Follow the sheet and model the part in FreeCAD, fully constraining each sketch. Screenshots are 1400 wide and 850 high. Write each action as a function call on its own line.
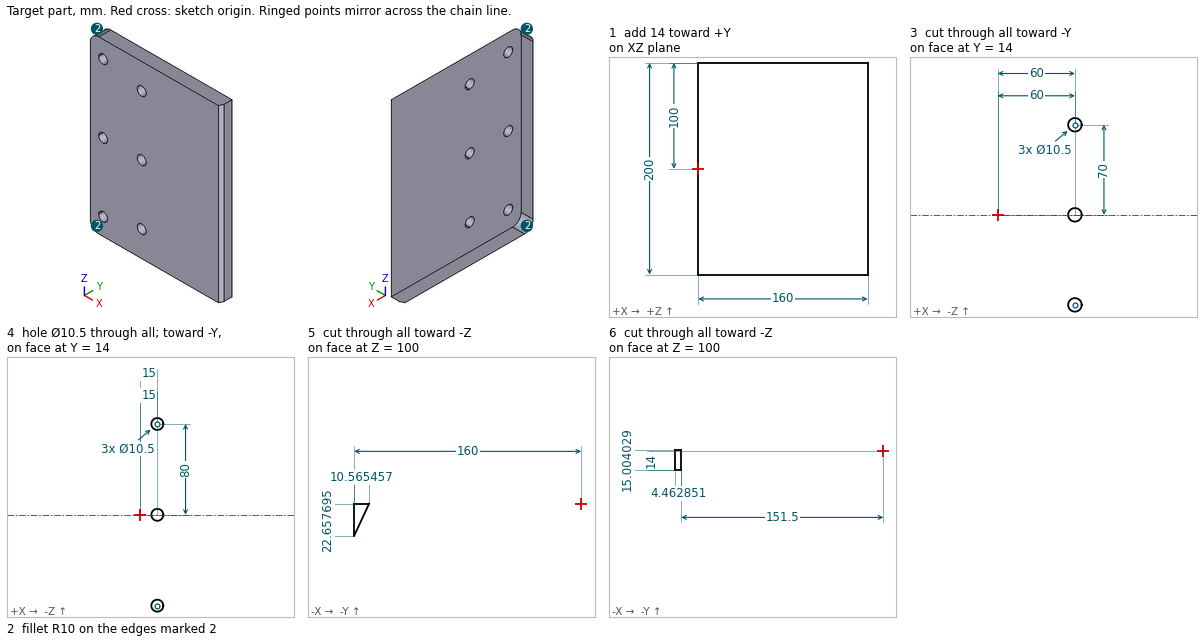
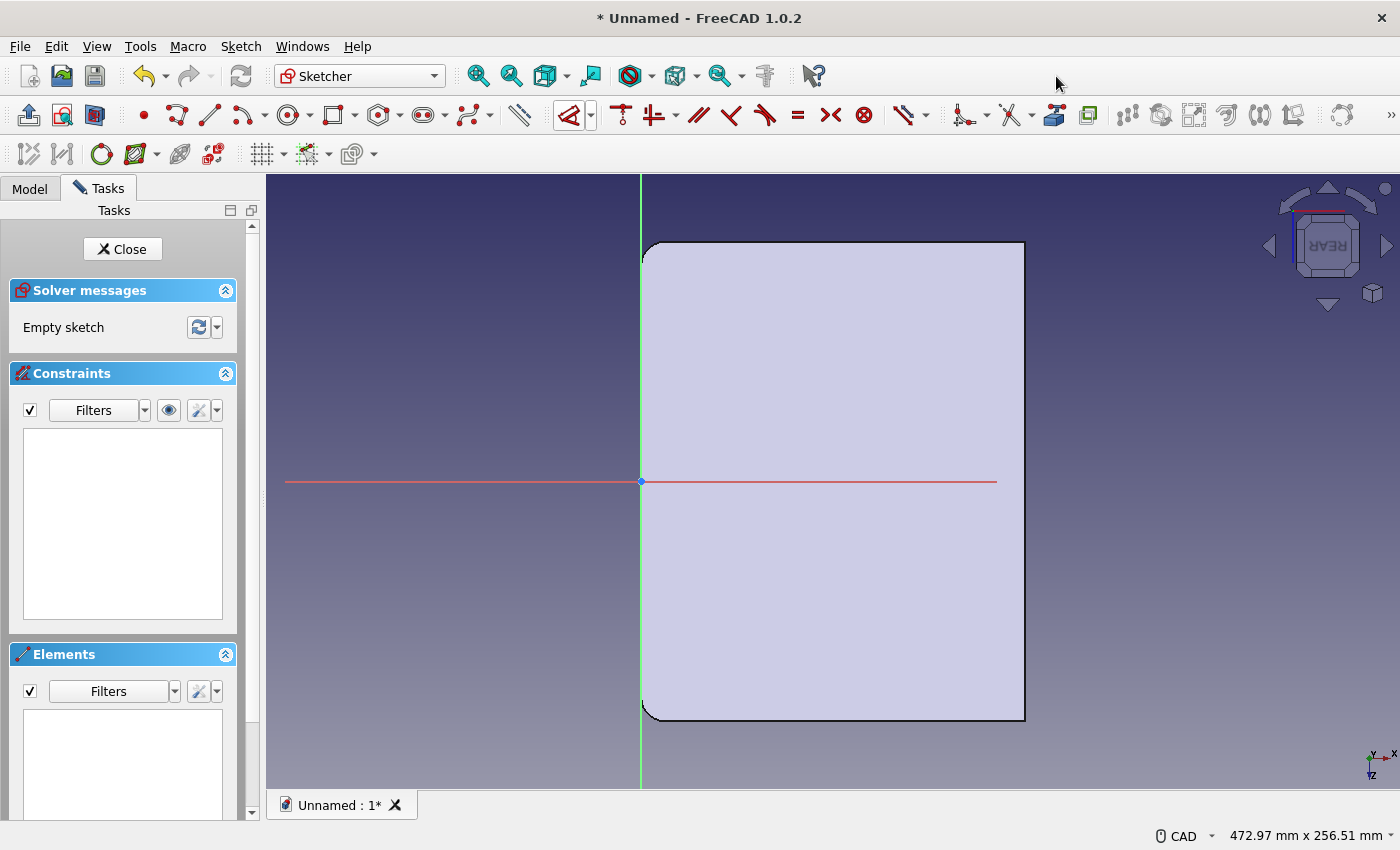
click(288, 116)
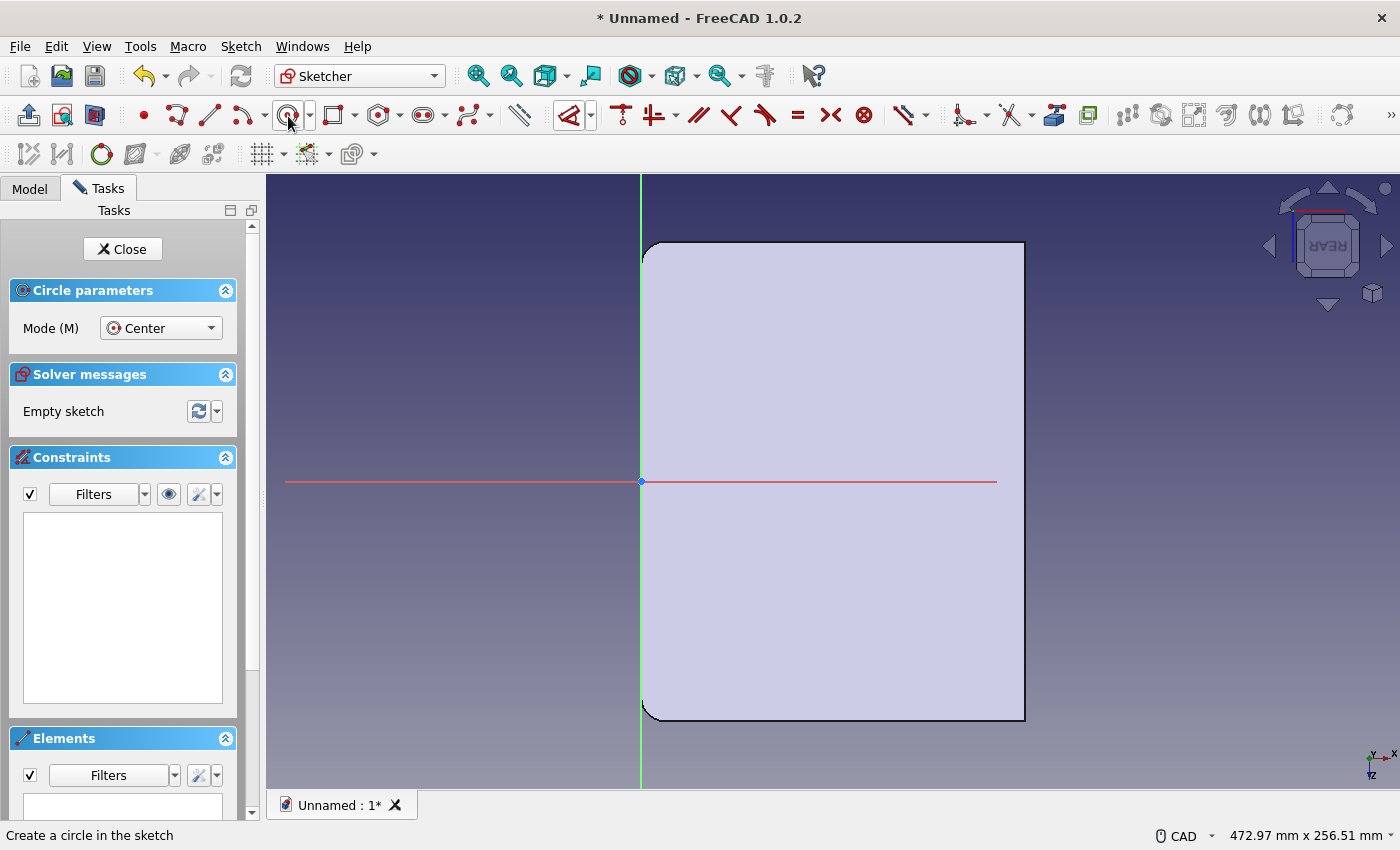
scroll(785, 314, up, 3)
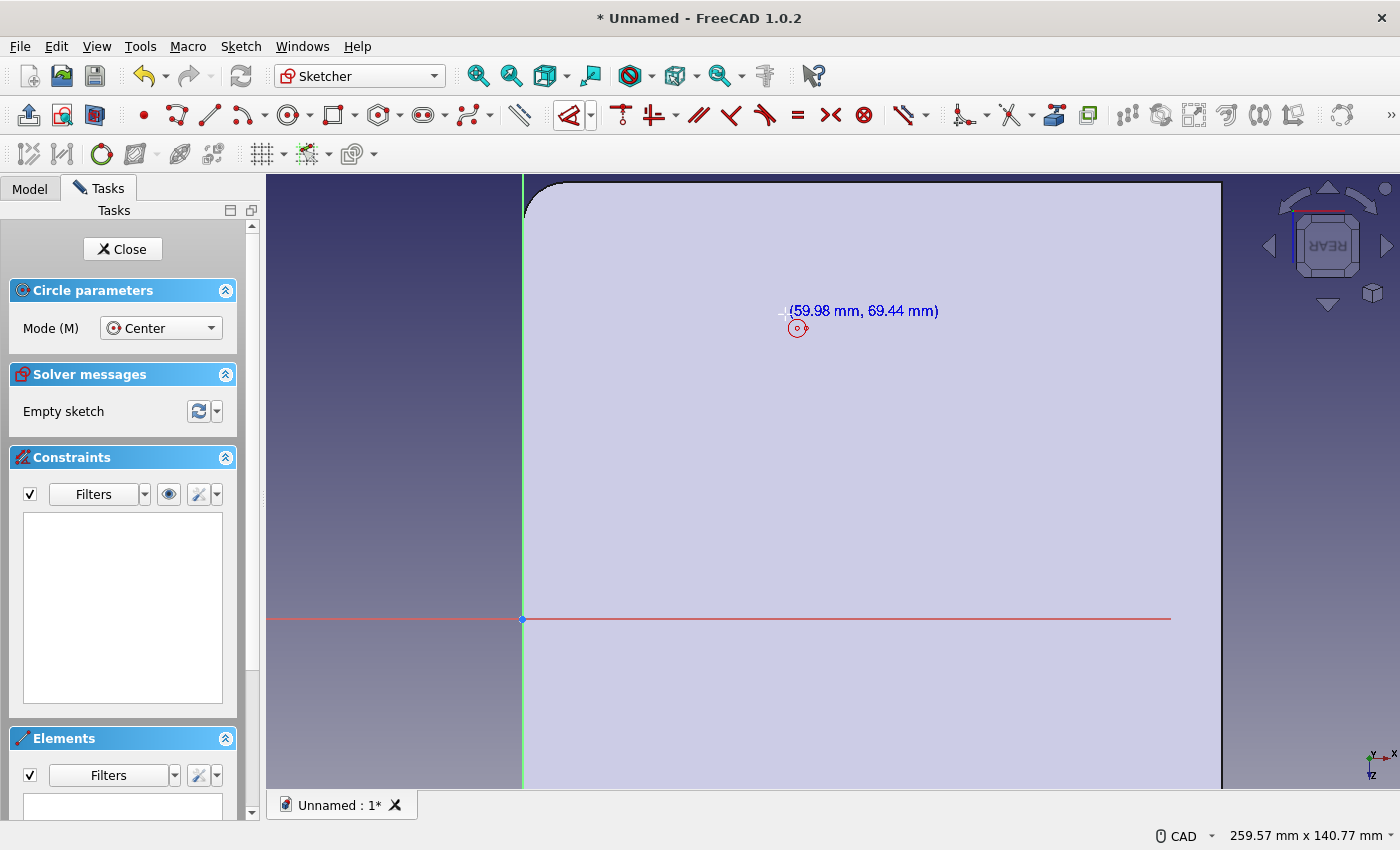
click(785, 313)
click(801, 297)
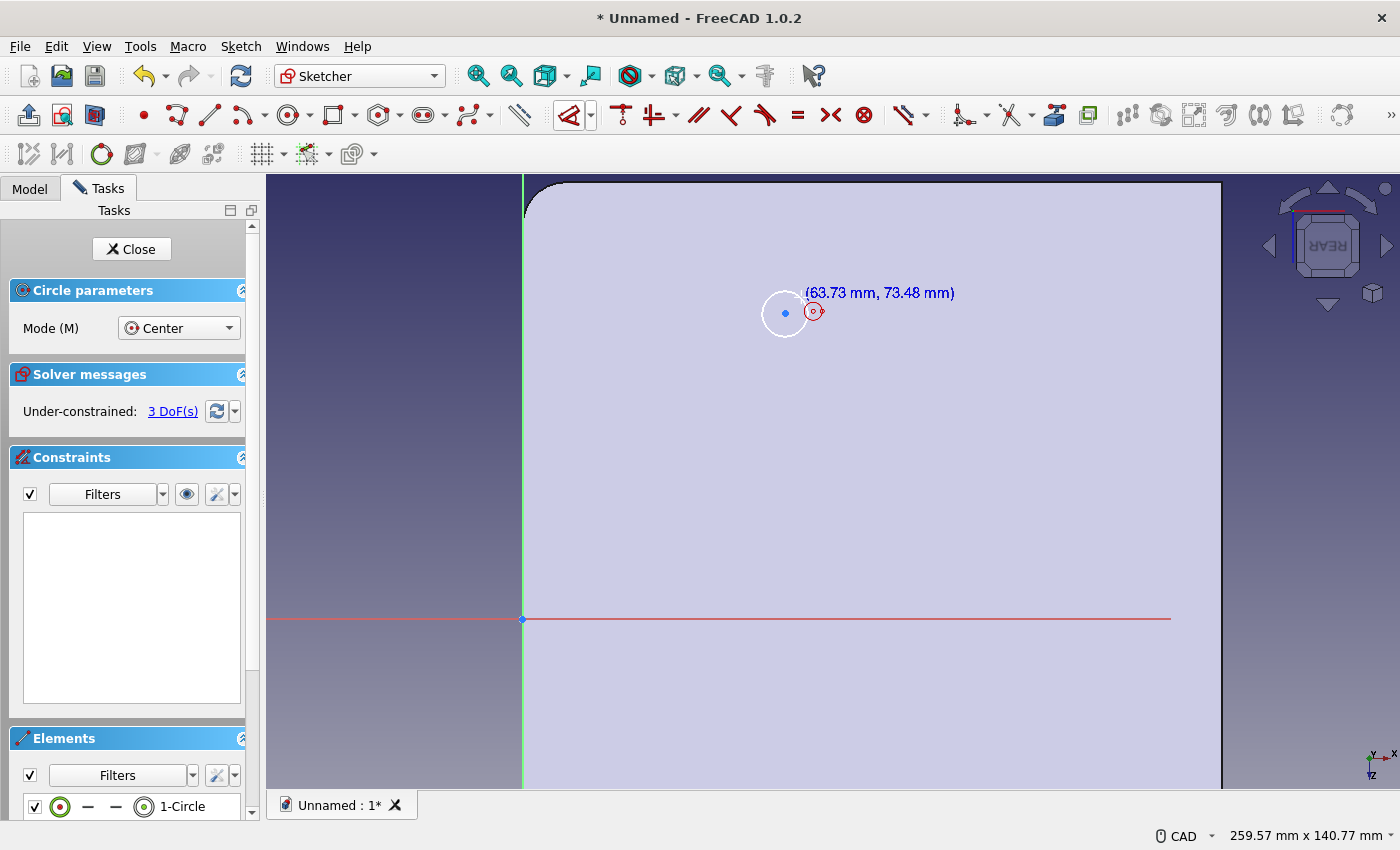
scroll(885, 314, down, 3)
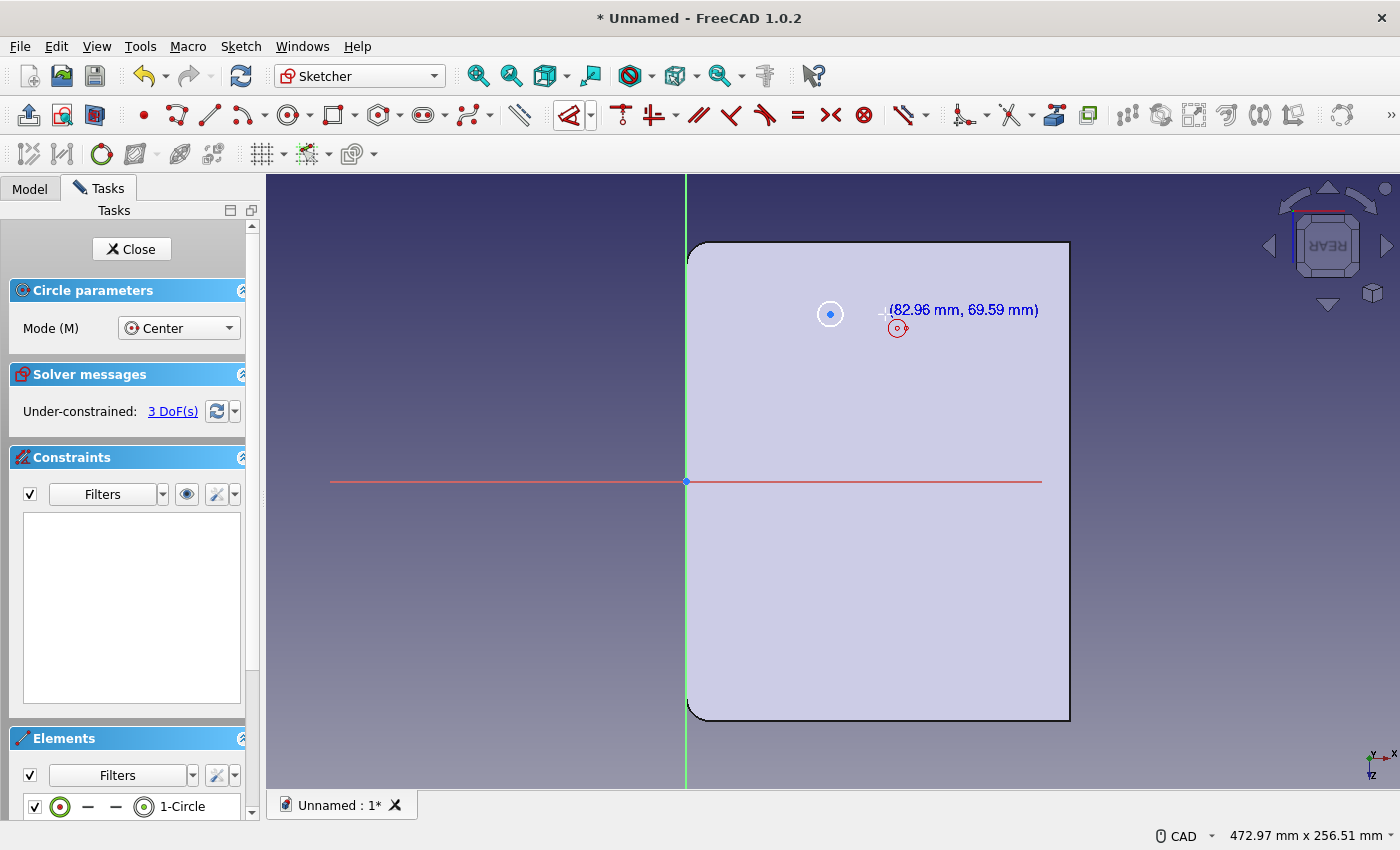
scroll(830, 649, up, 3)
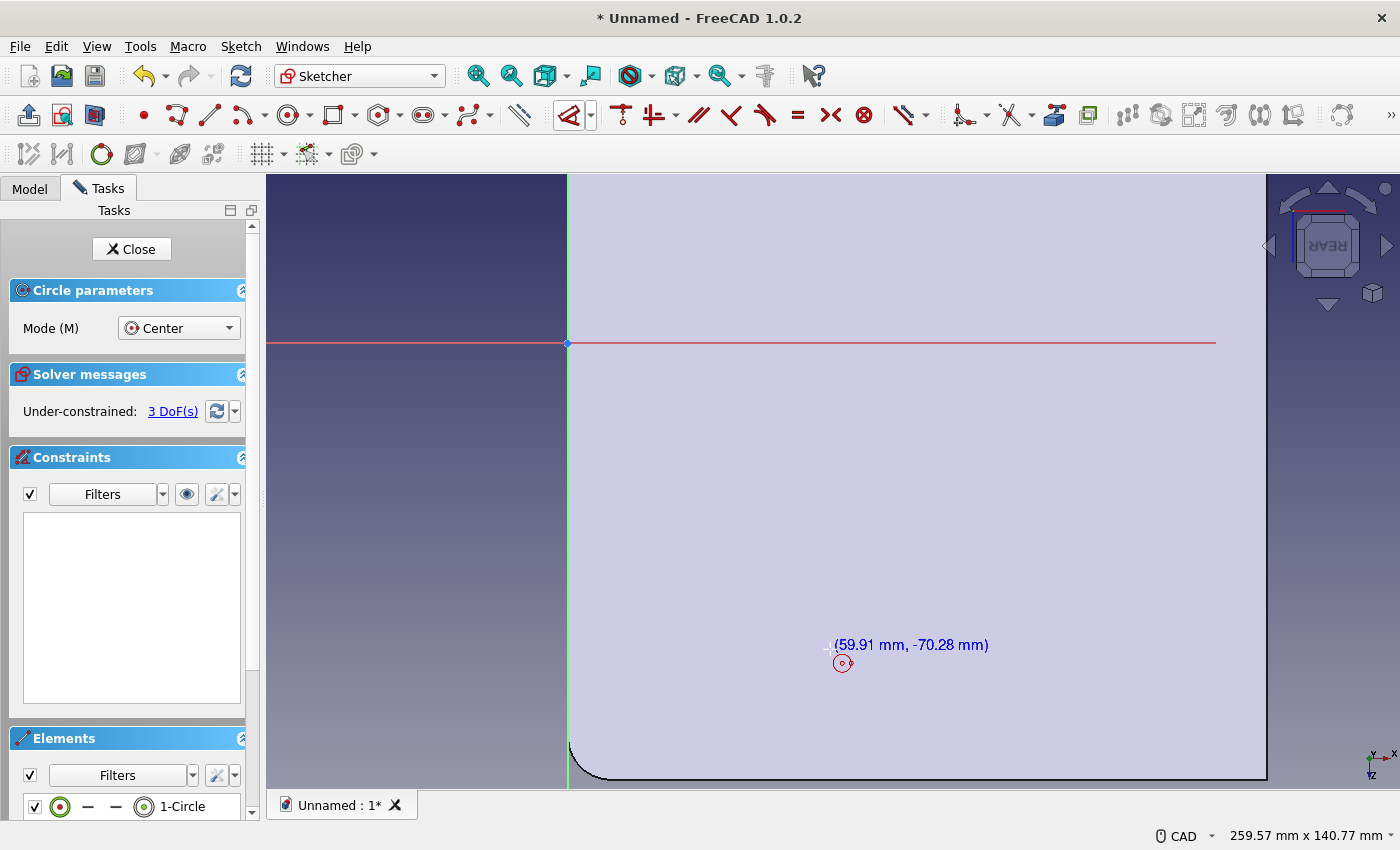
click(830, 649)
click(846, 633)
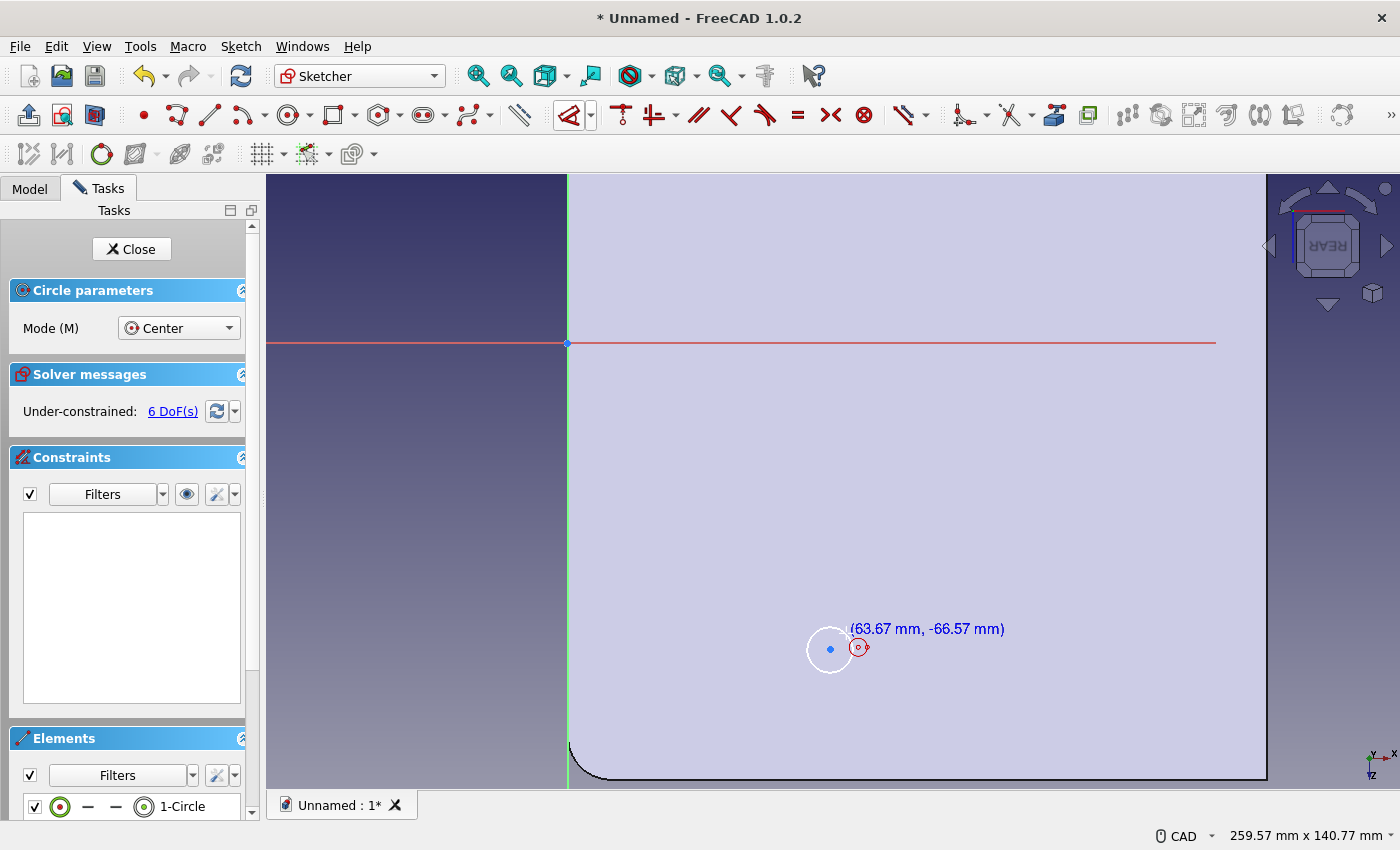
click(830, 343)
click(846, 327)
key(Escape)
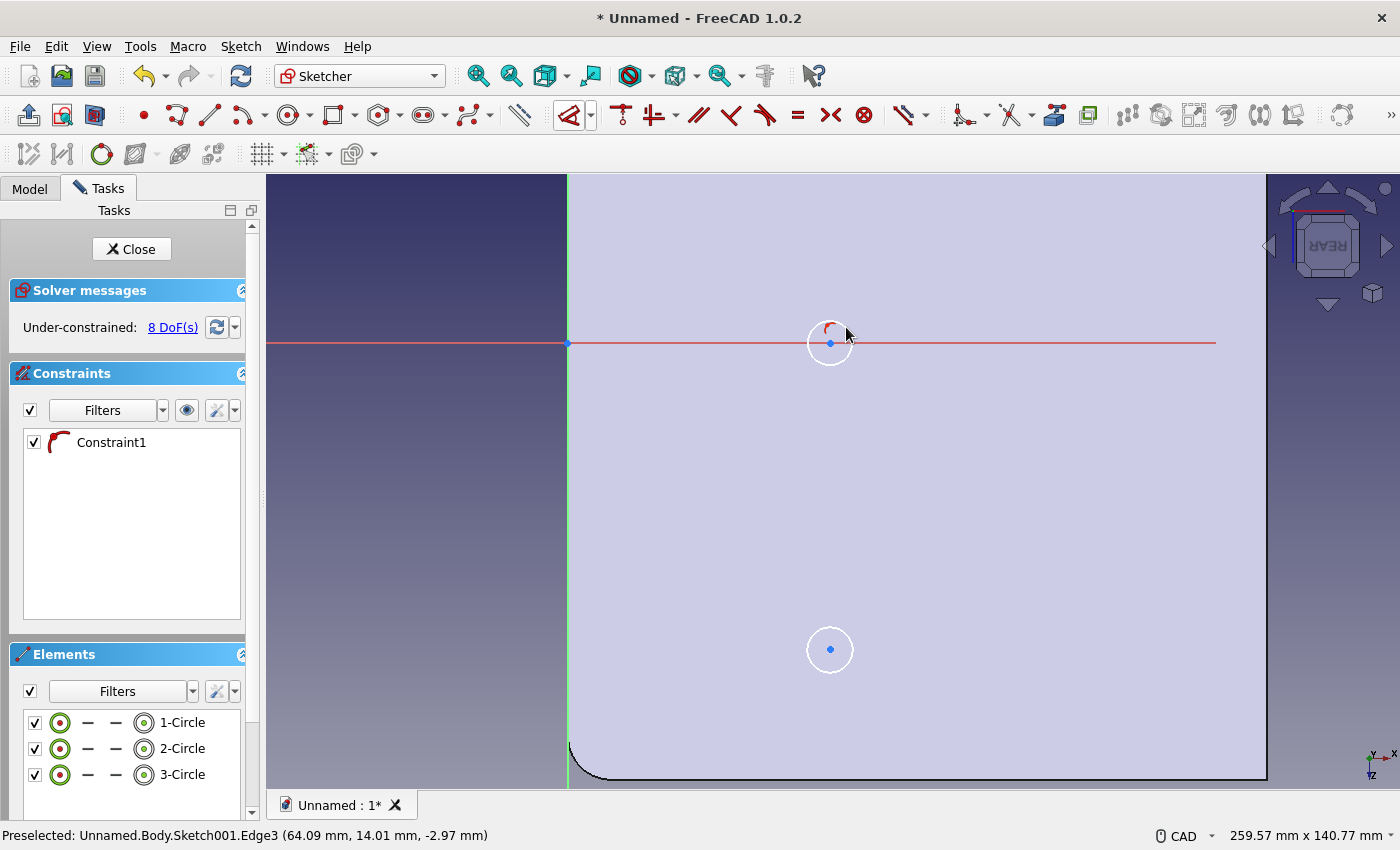
scroll(830, 650, down, 3)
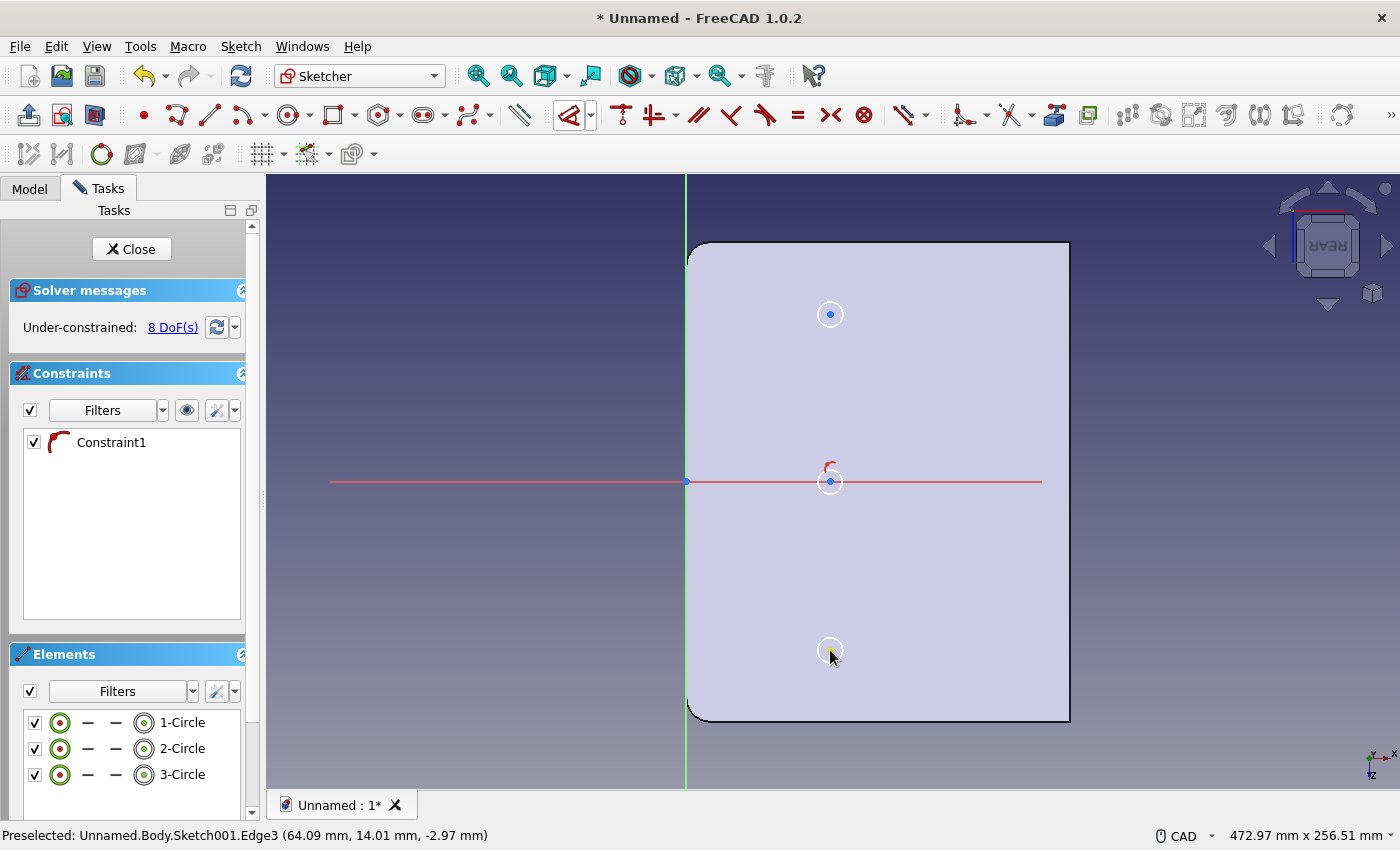
click(839, 306)